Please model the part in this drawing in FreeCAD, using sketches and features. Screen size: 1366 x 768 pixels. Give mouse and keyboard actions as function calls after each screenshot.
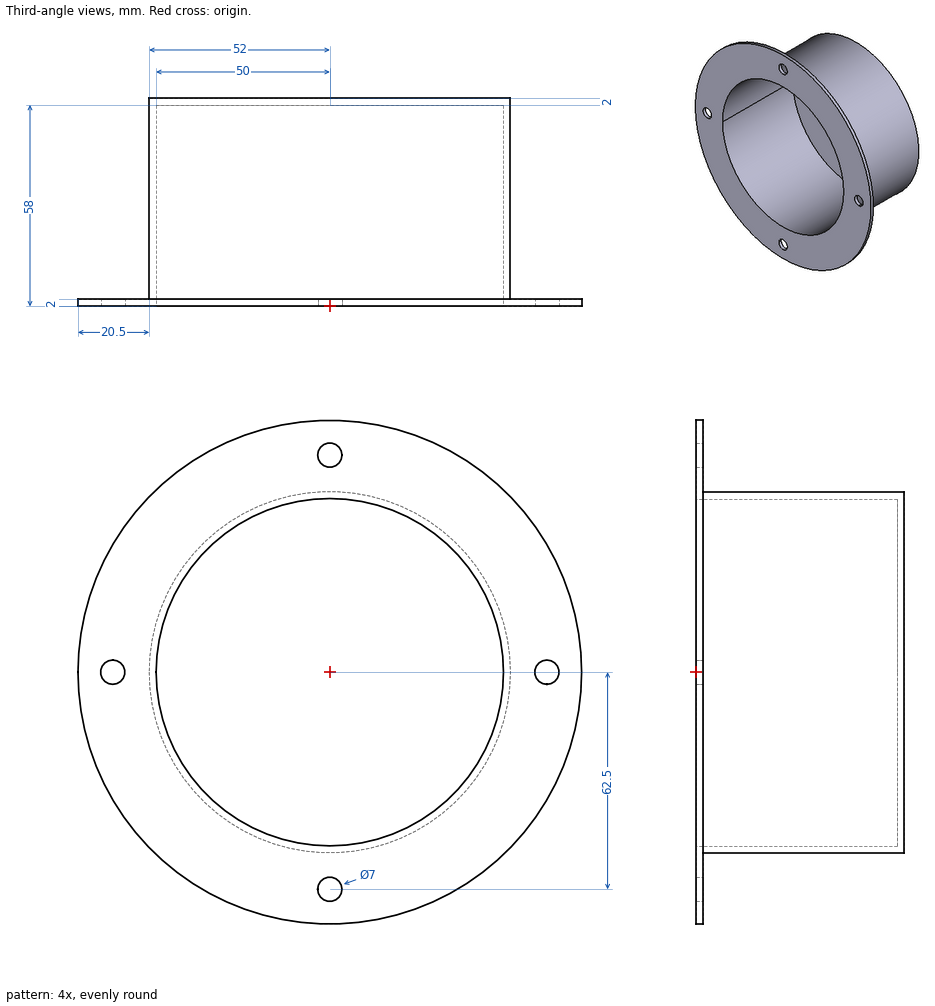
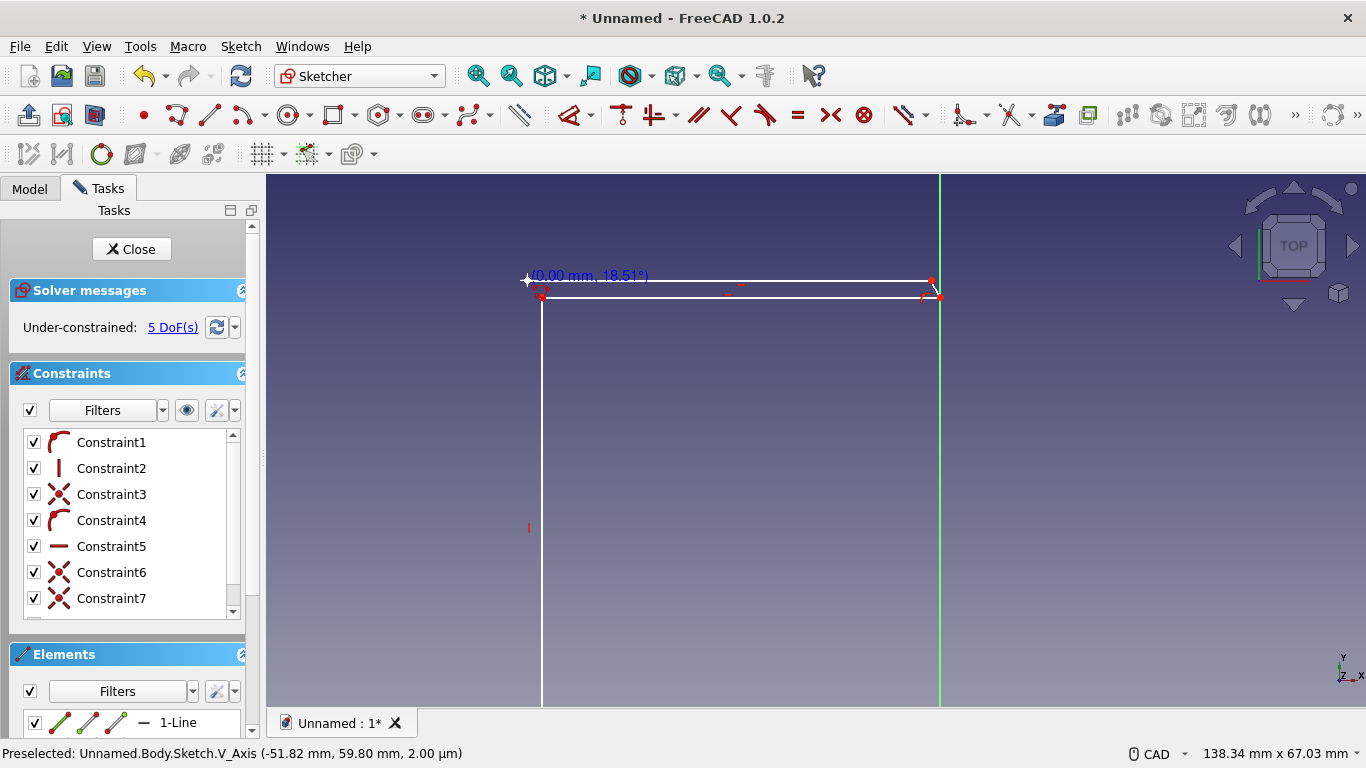
scroll(942, 281, down, 2)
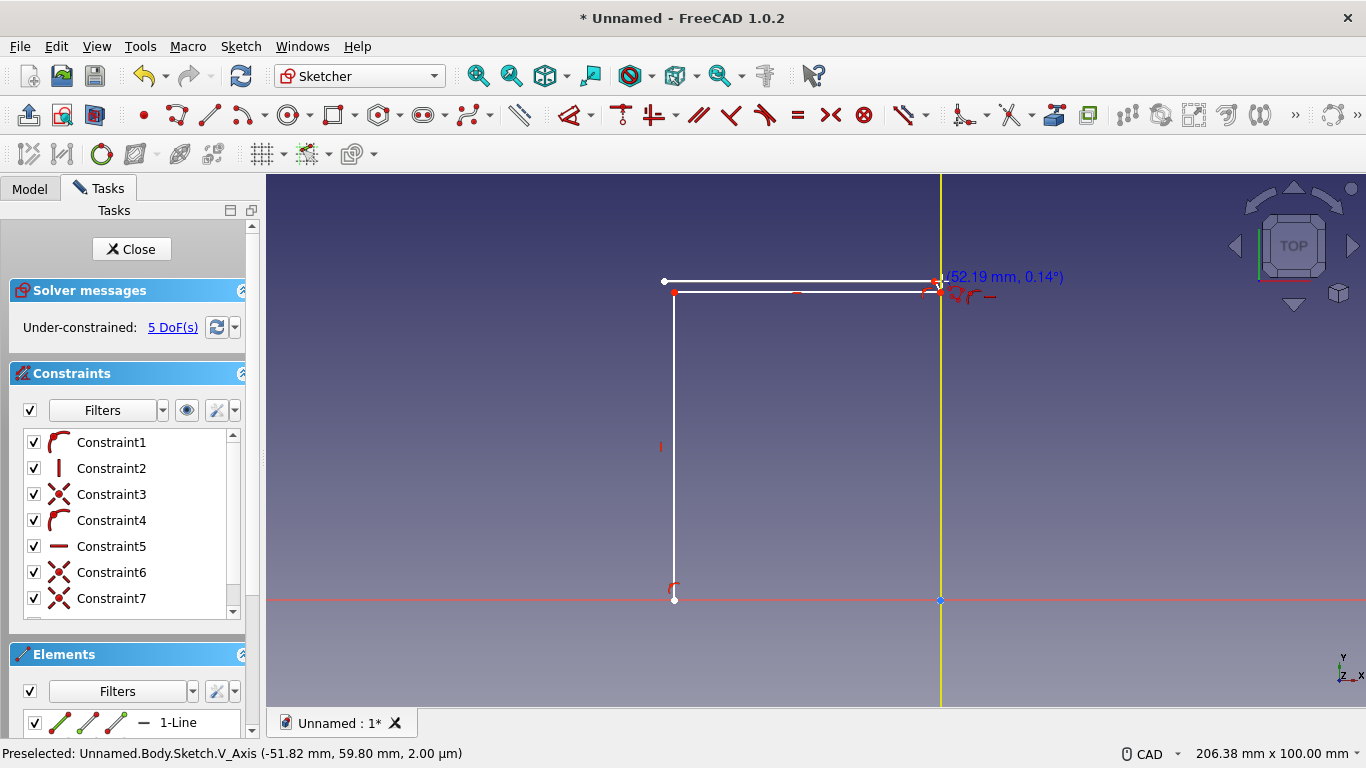
scroll(664, 590, up, 2)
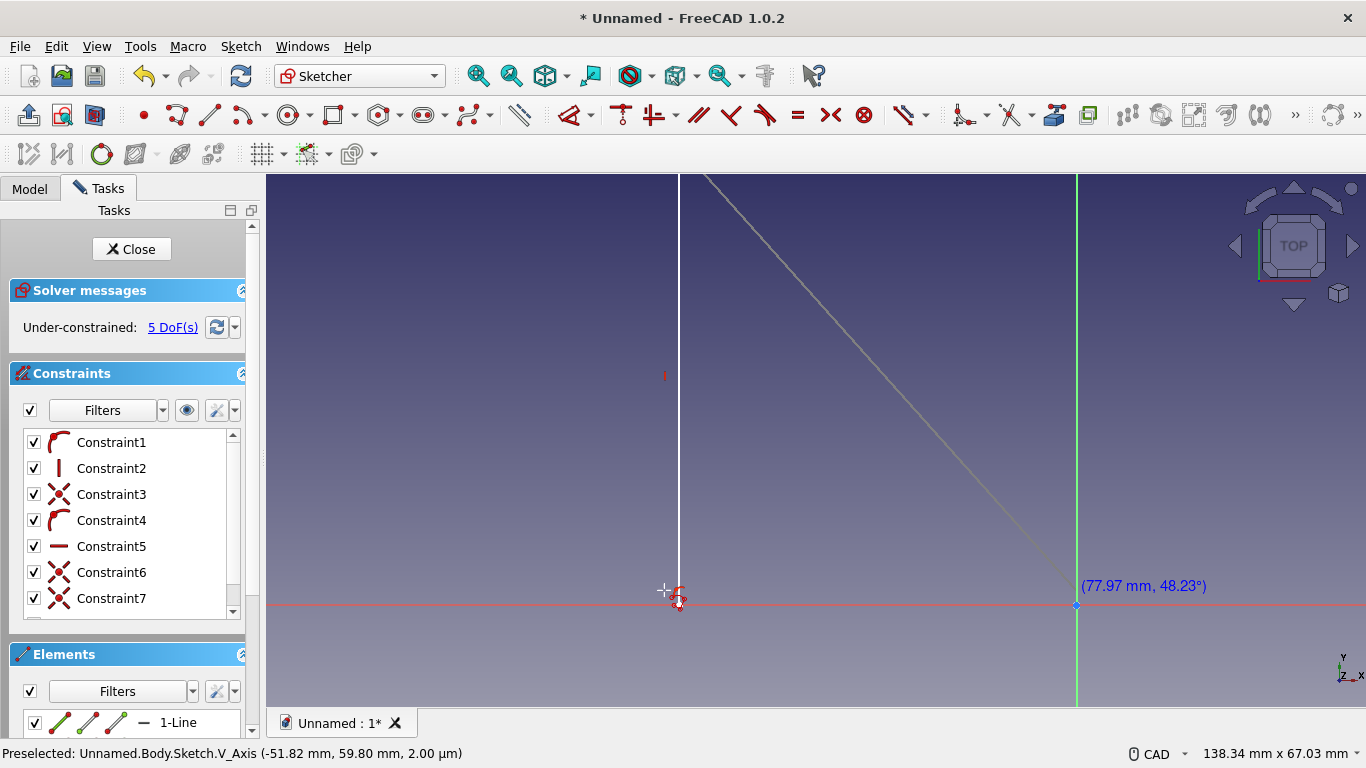
click(664, 589)
click(500, 589)
click(500, 596)
click(679, 605)
key(Escape)
key(Escape)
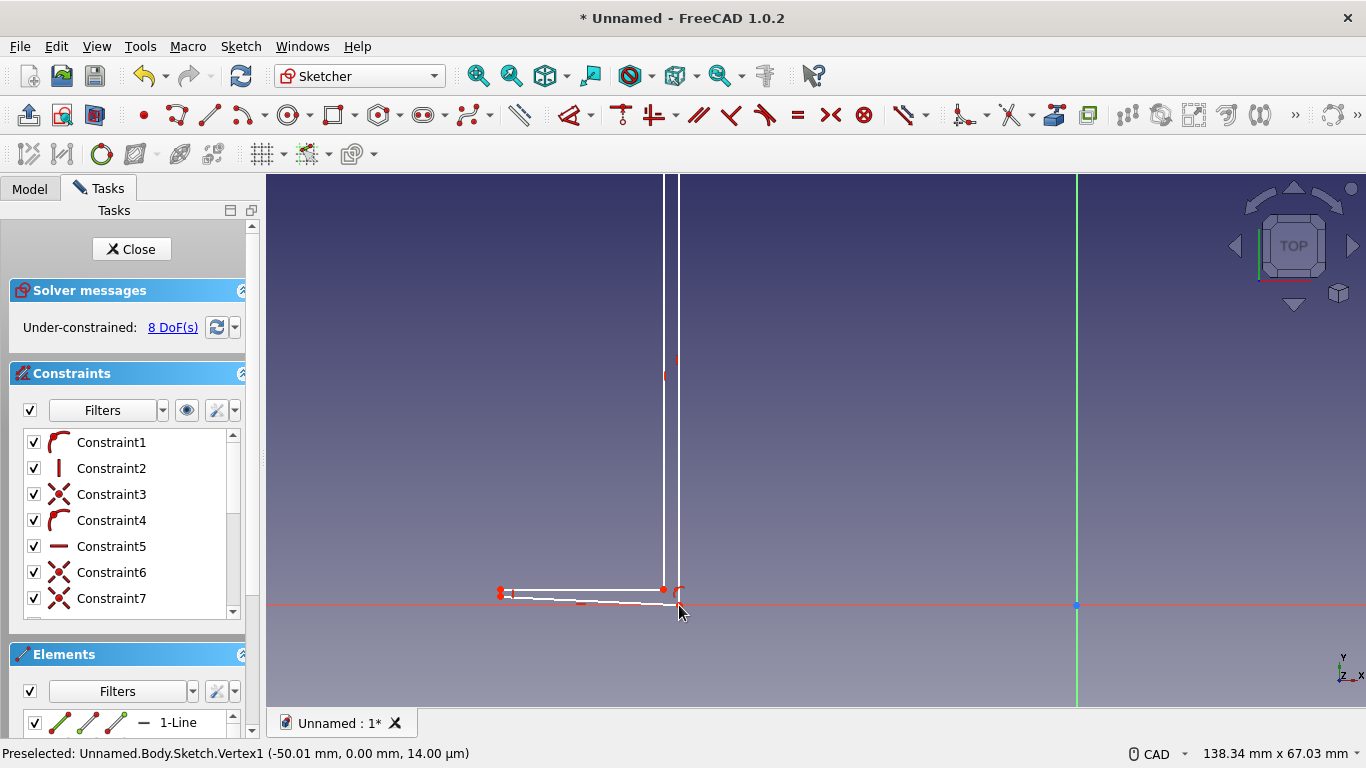
scroll(664, 591, down, 2)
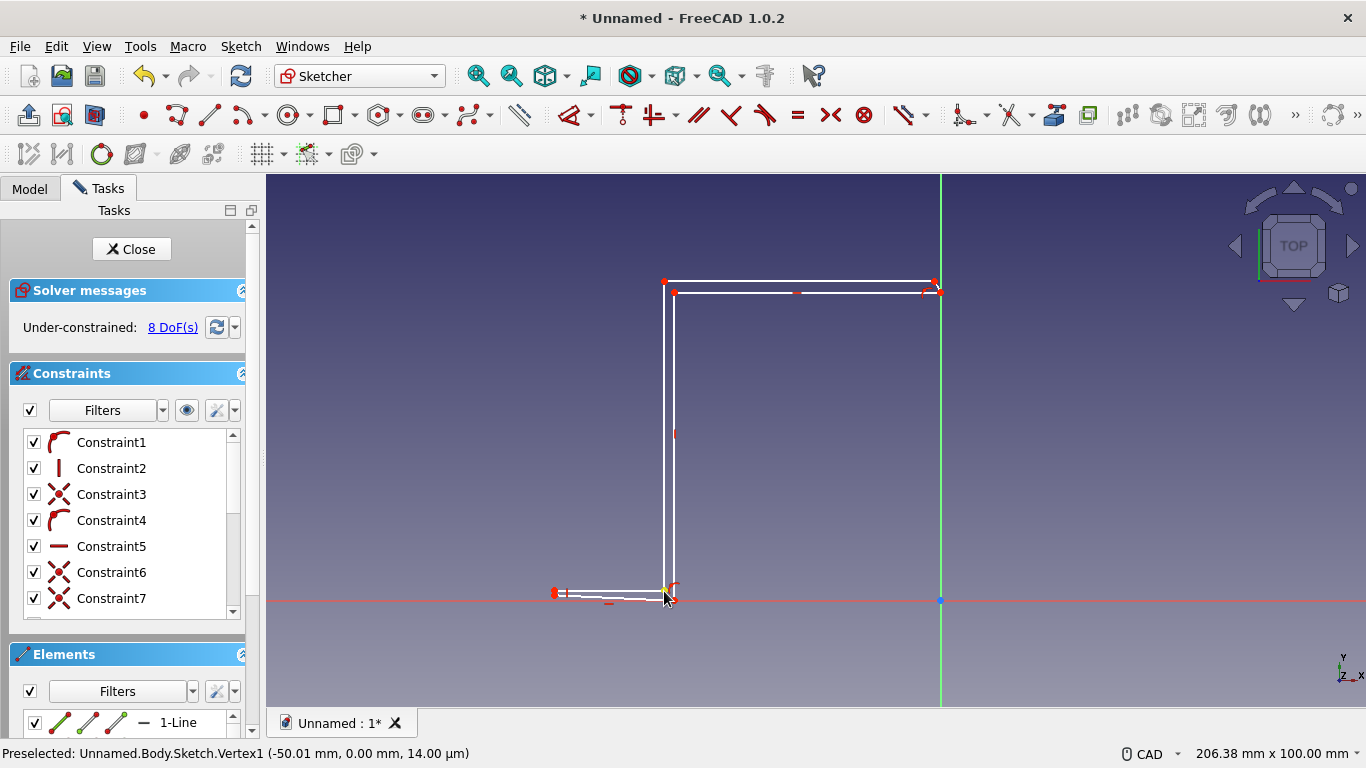
scroll(938, 288, up, 6)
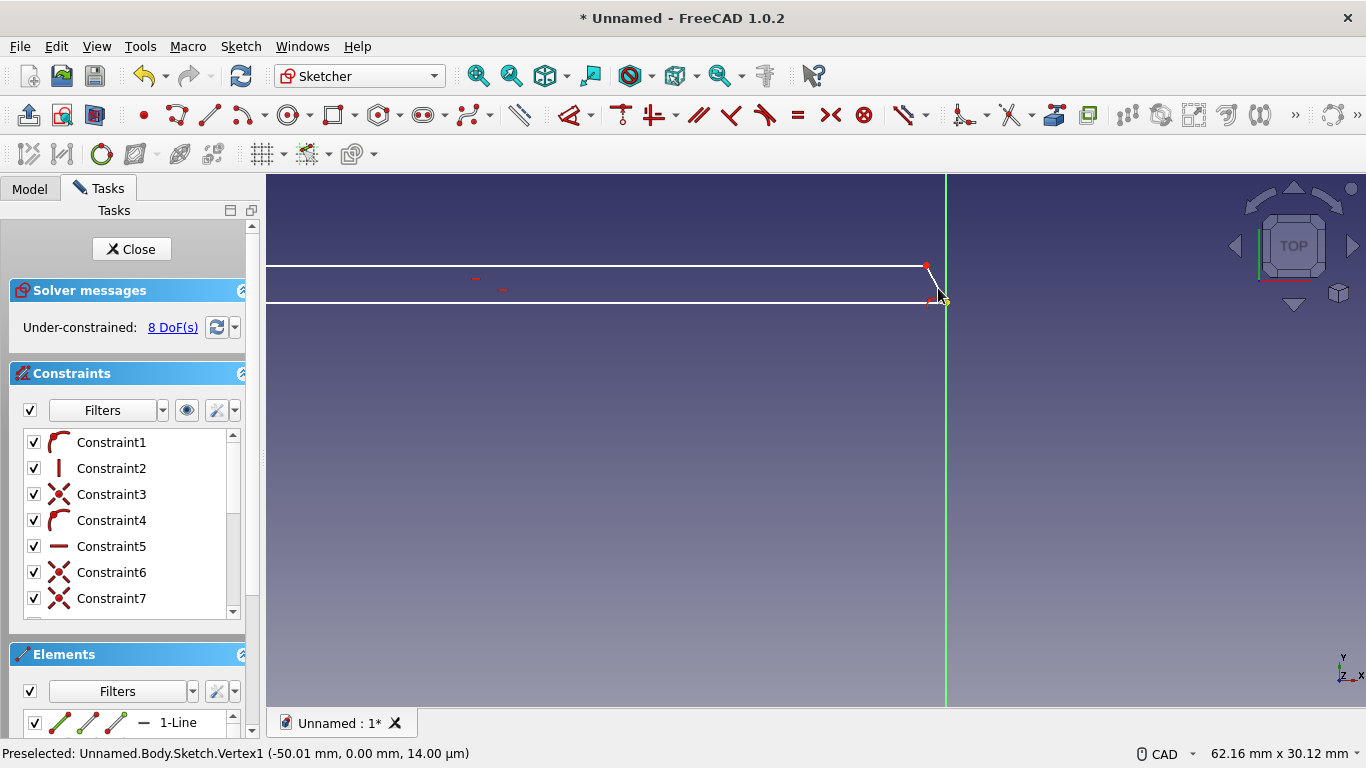
click(938, 288)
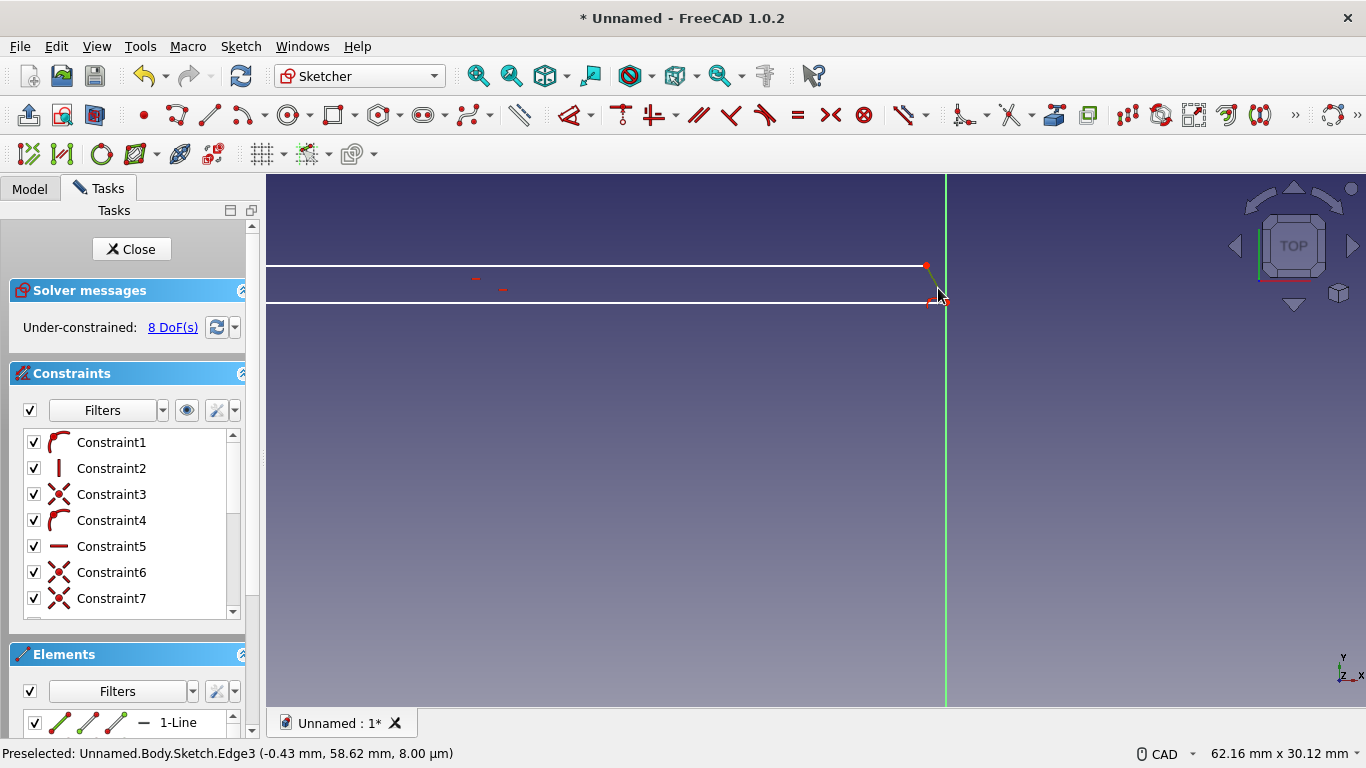
key(v)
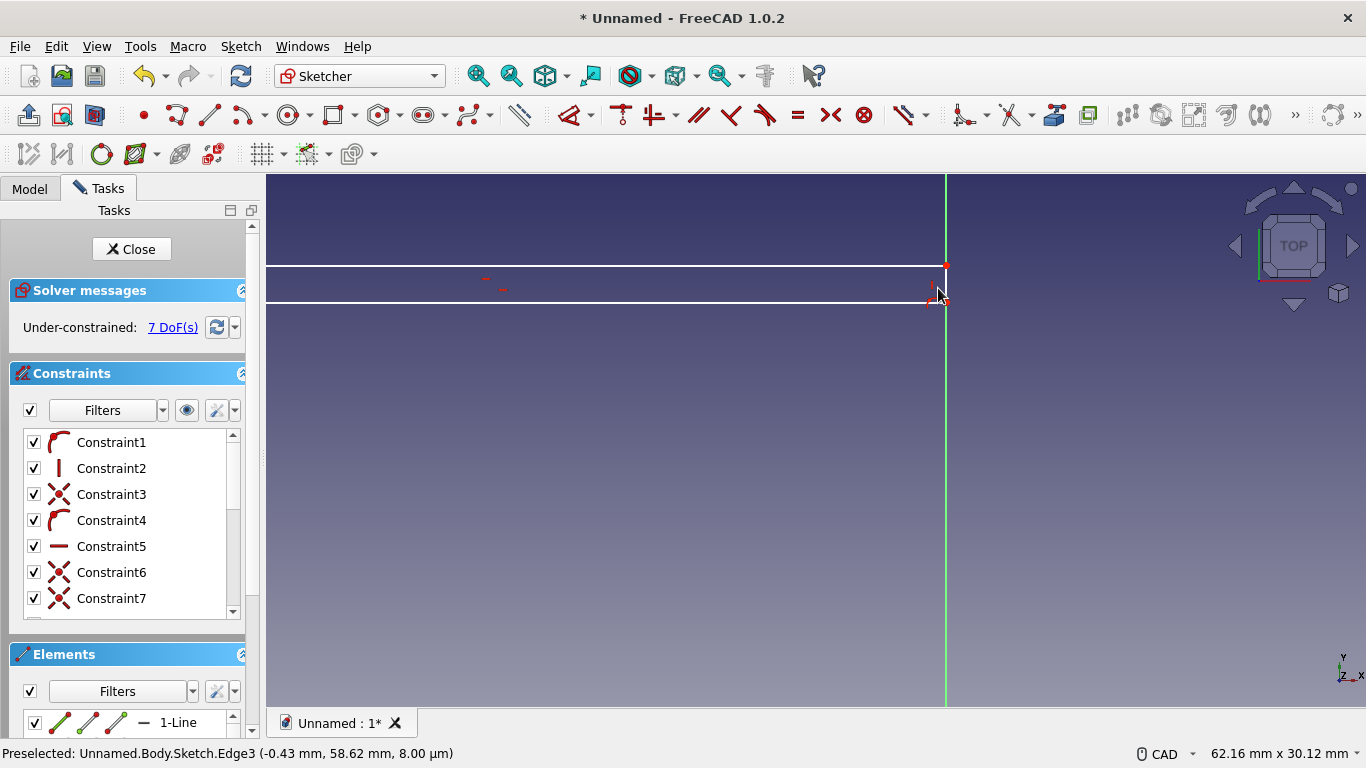
scroll(938, 288, down, 6)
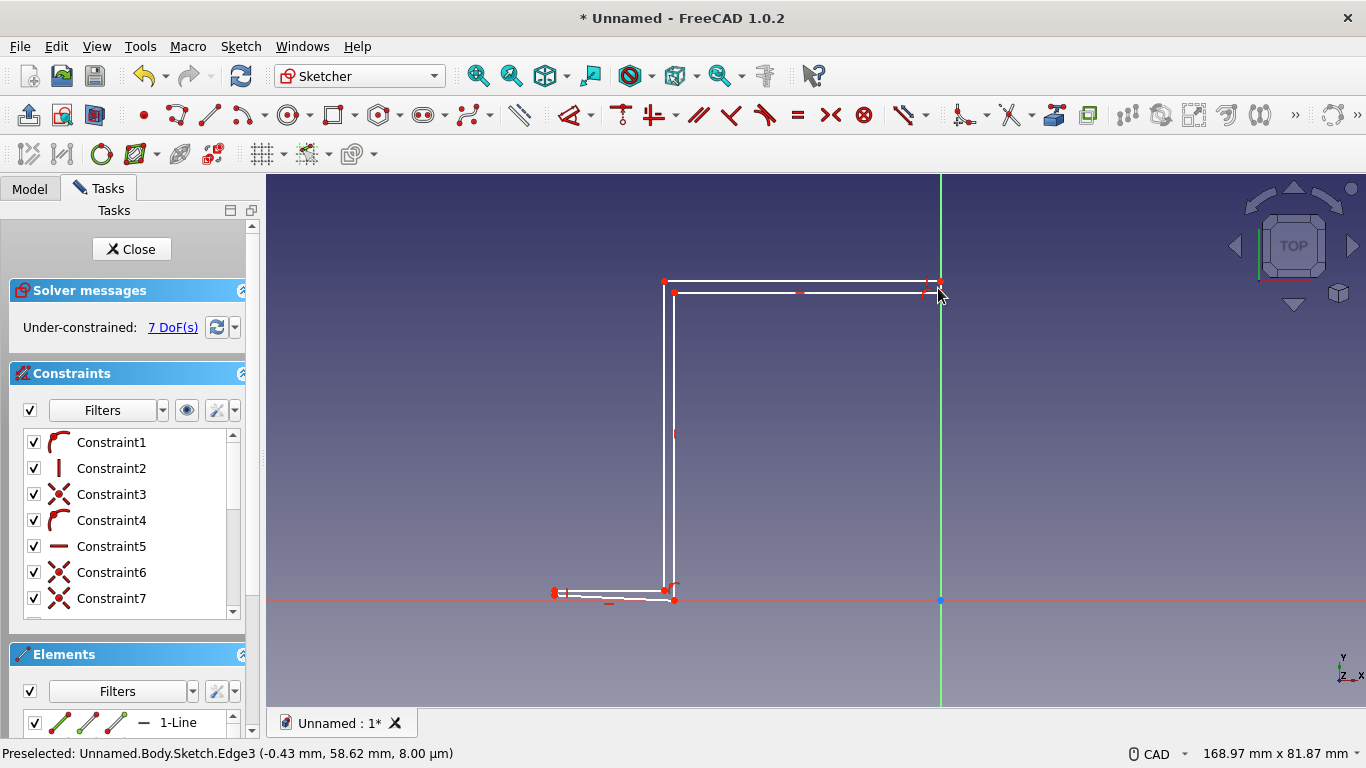
scroll(590, 597, up, 7)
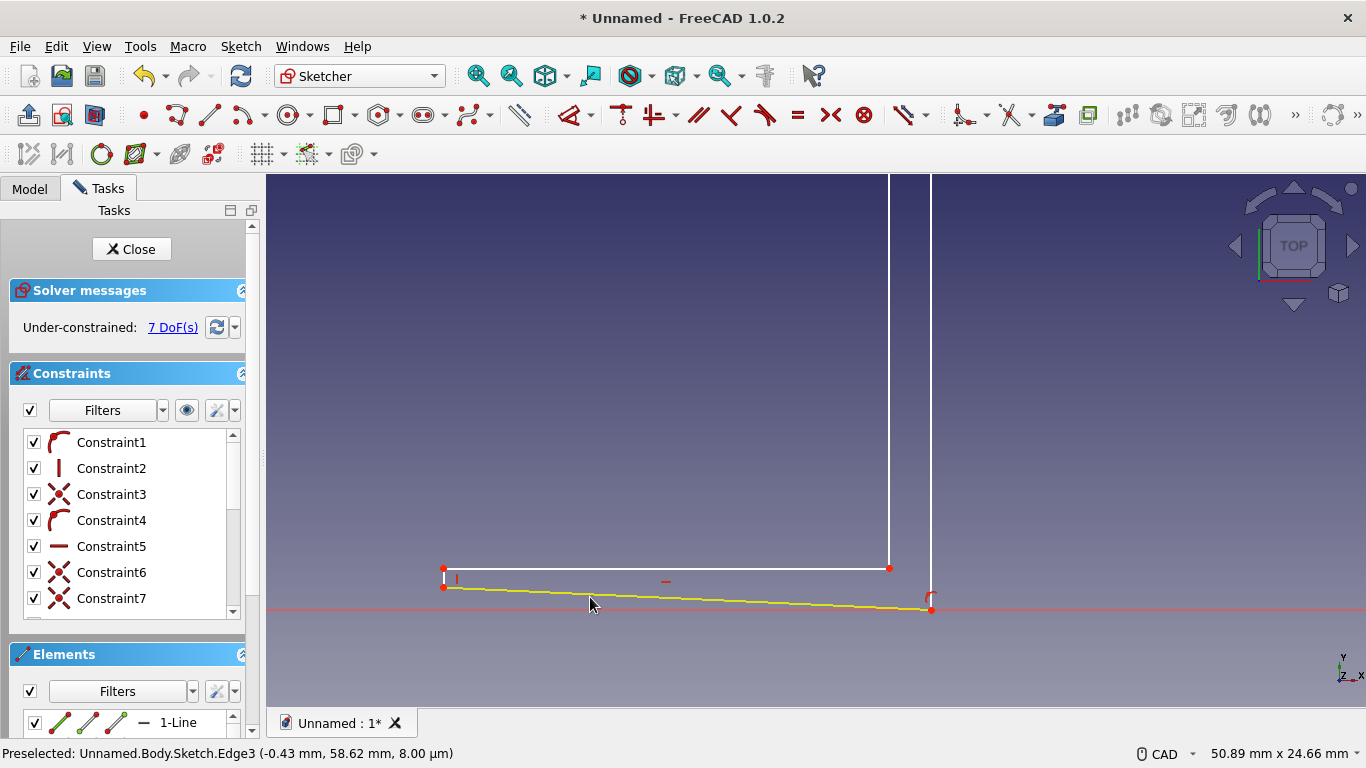
click(590, 594)